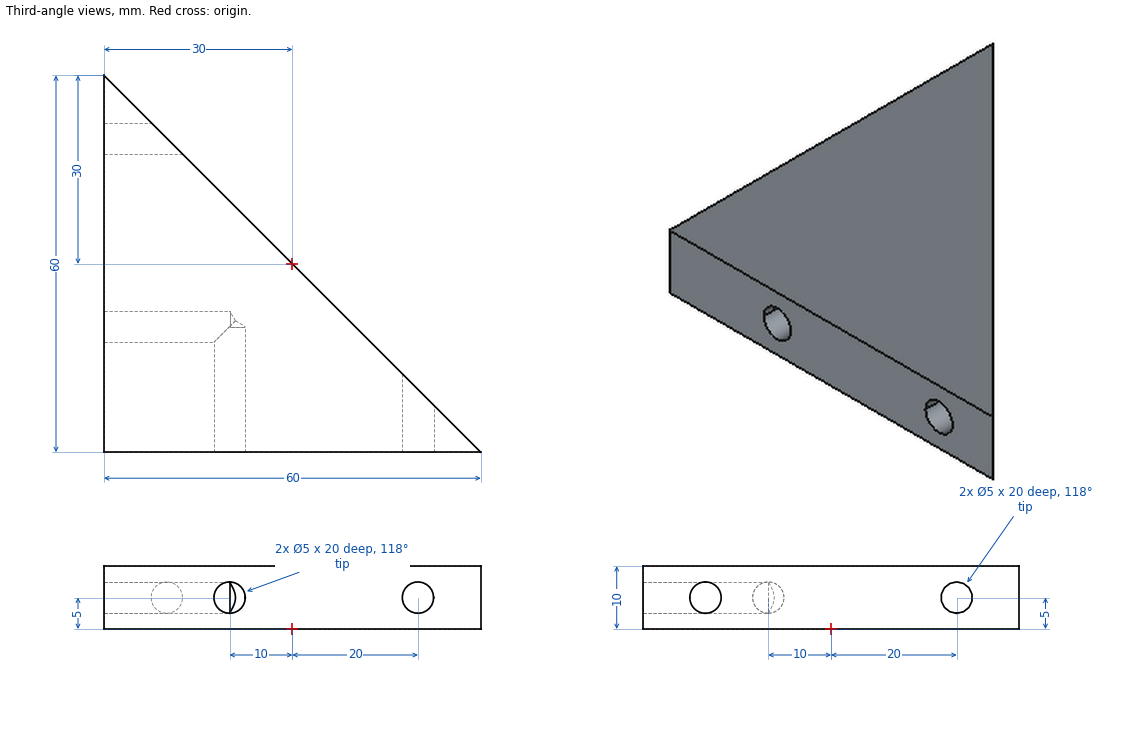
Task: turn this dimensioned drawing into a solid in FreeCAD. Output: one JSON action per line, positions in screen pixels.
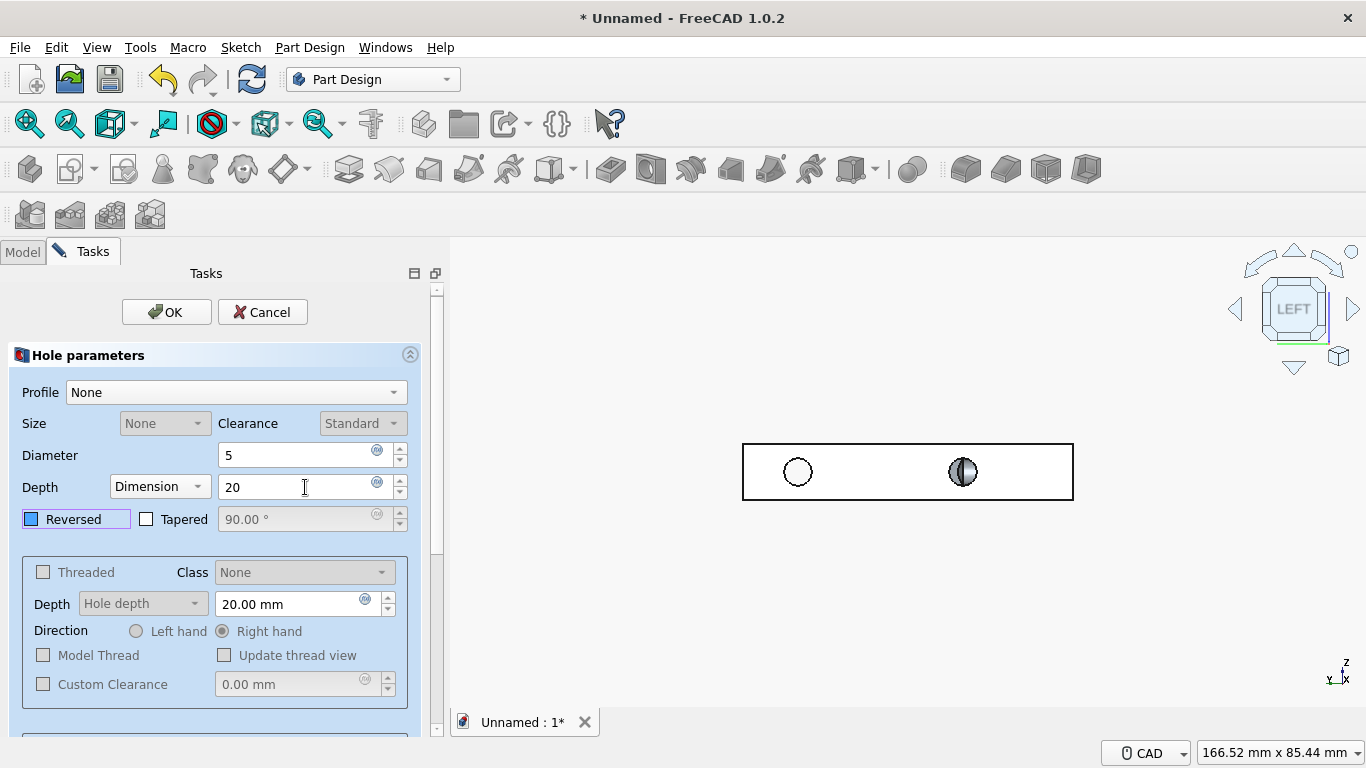
{"action": "left_click", "coordinate": [167, 312]}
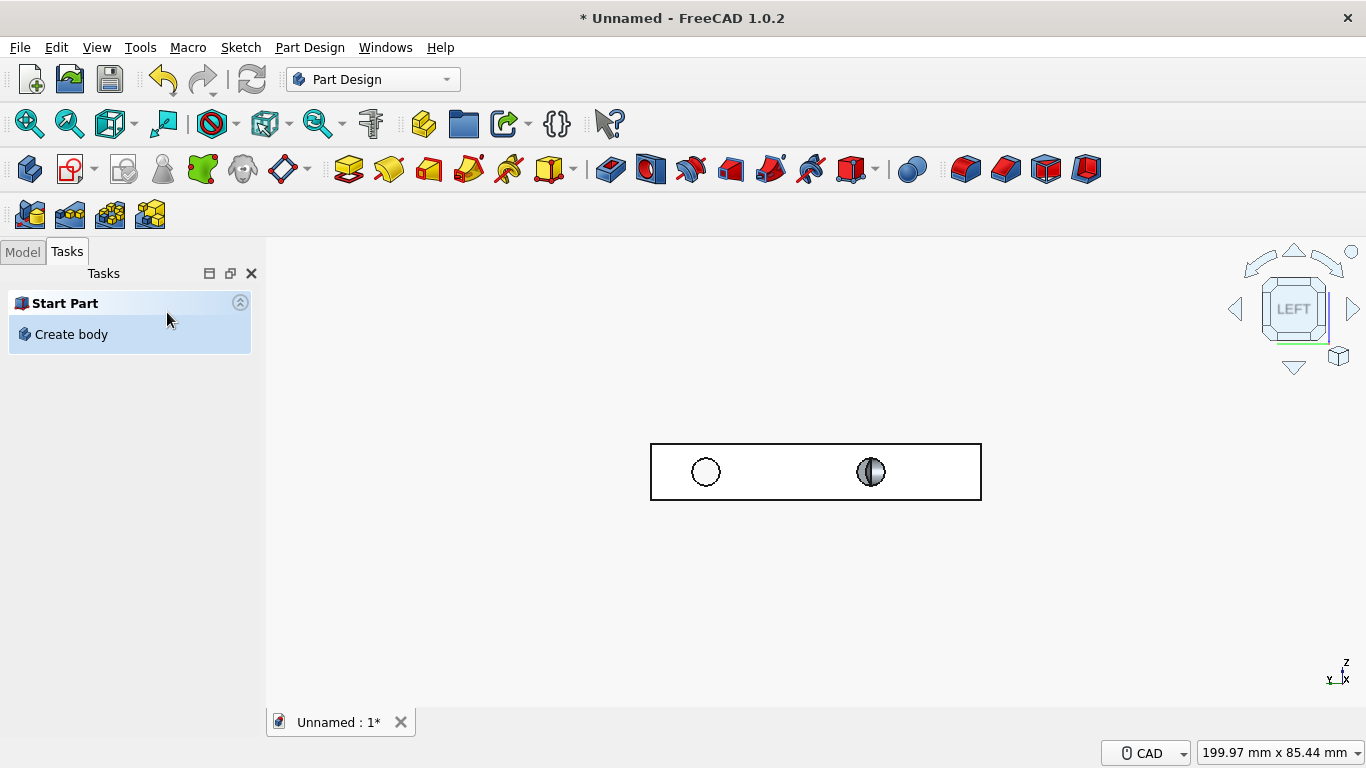
{"action": "key", "text": "0"}